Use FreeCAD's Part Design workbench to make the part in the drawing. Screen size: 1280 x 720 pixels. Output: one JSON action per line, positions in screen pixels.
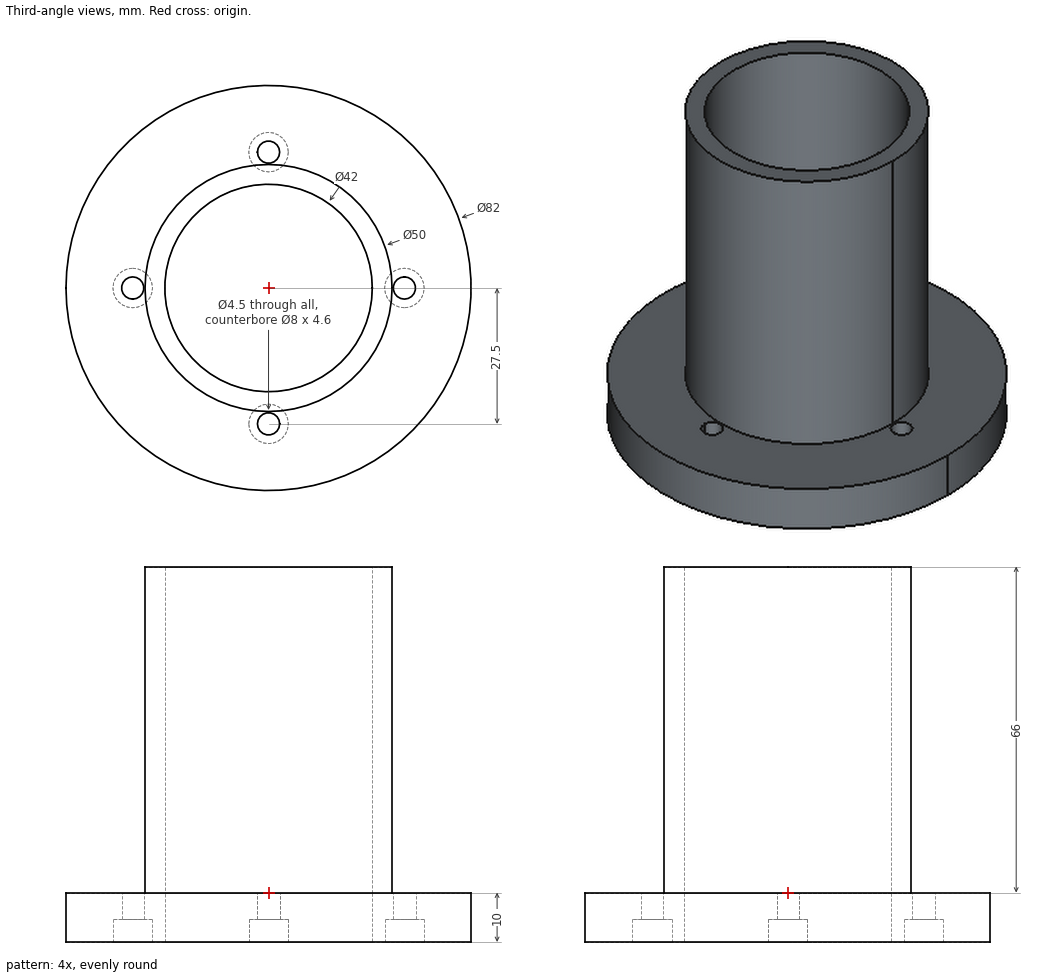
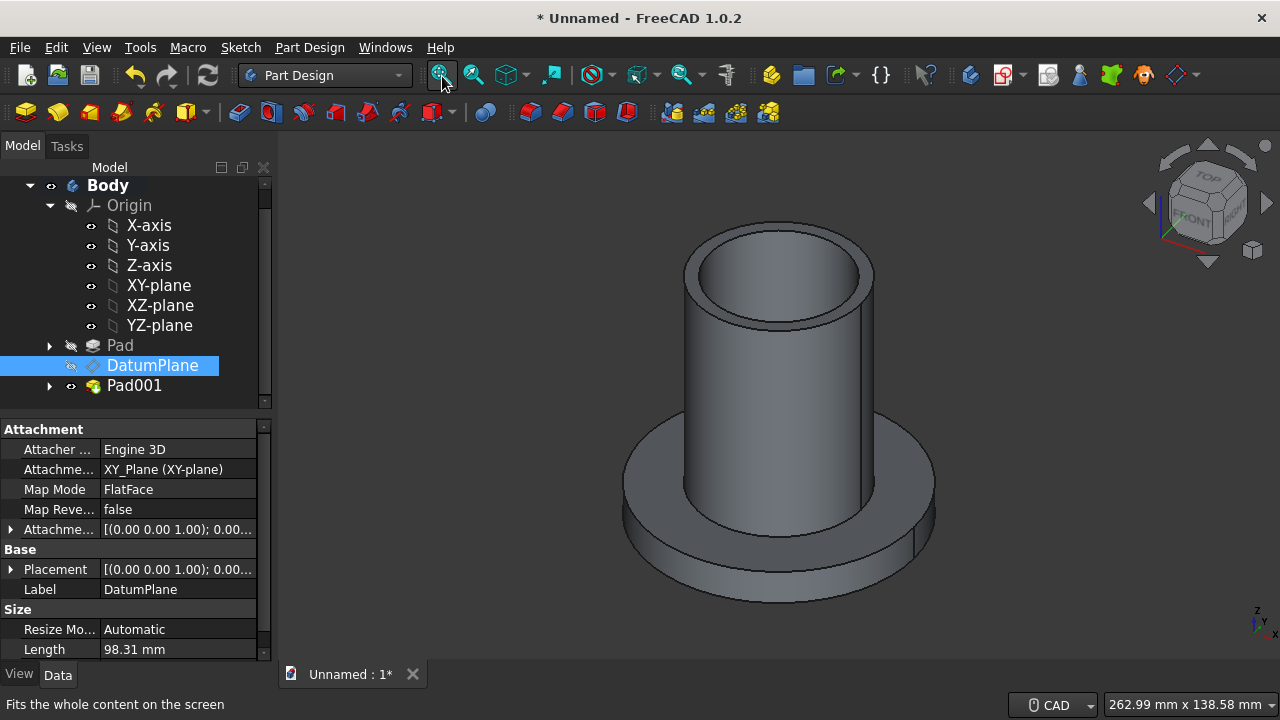
{"action": "key", "text": "5"}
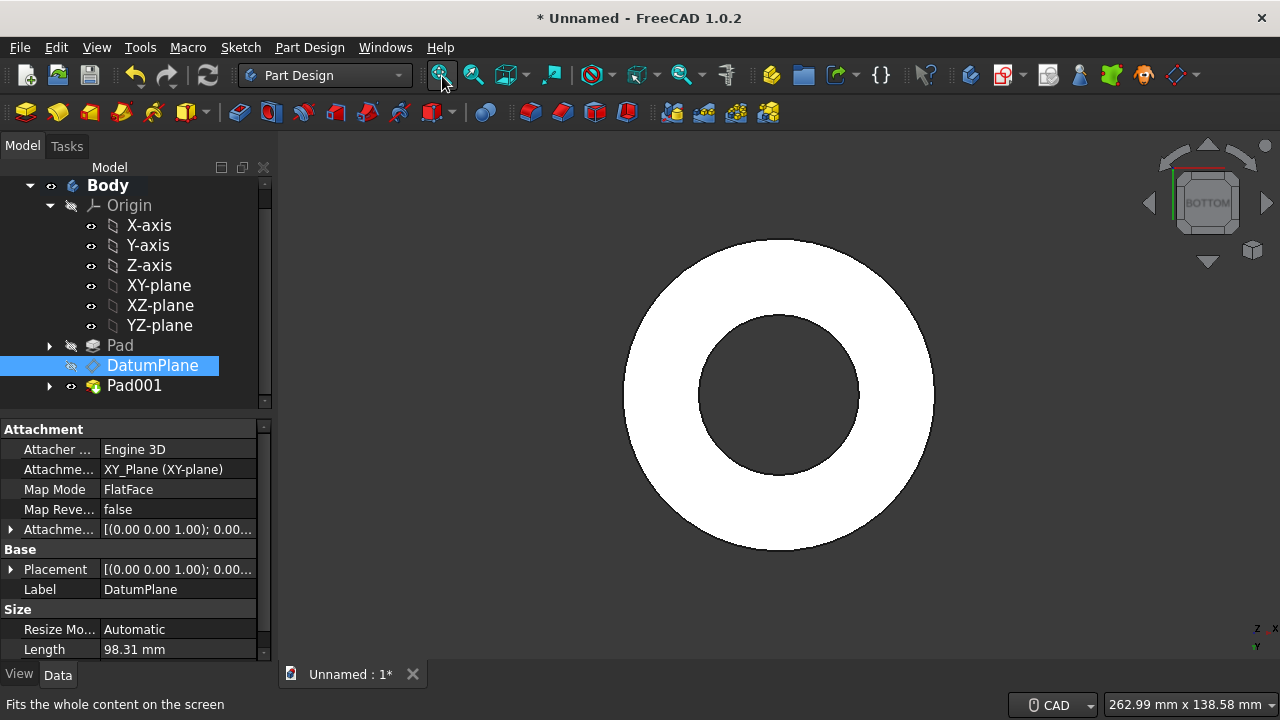
{"action": "left_click", "coordinate": [868, 305]}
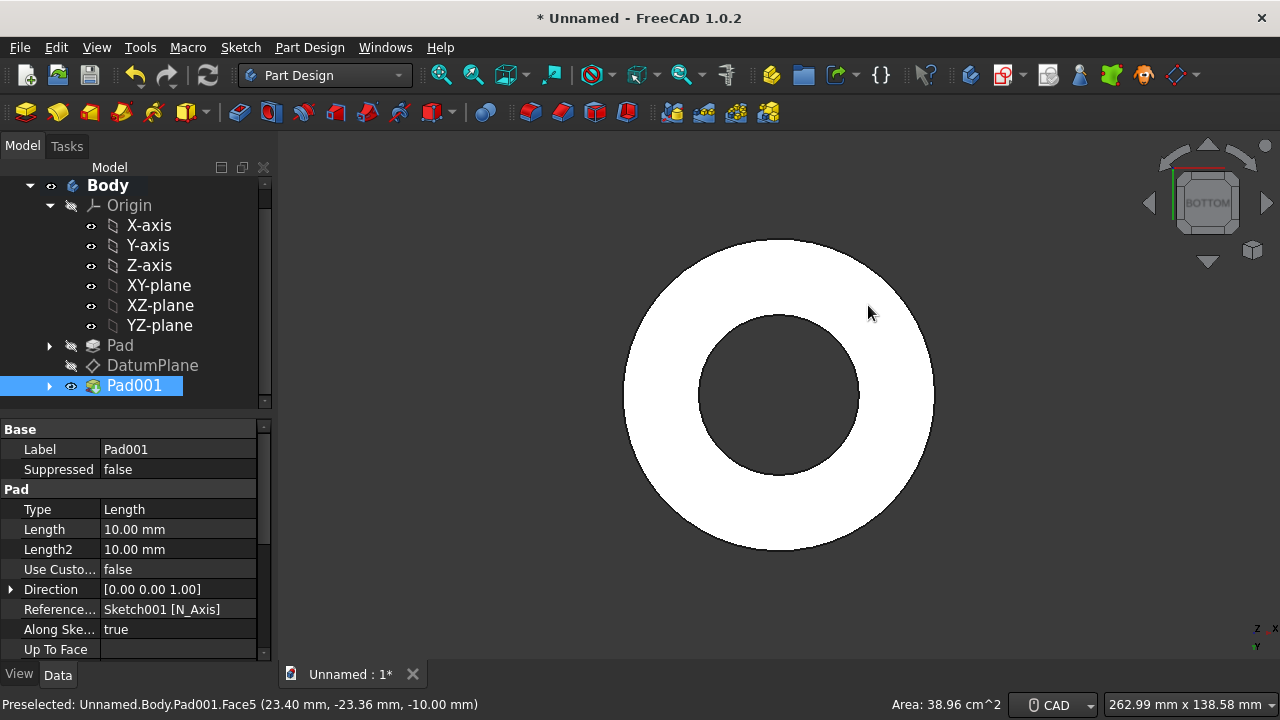
{"action": "left_click", "coordinate": [1004, 76]}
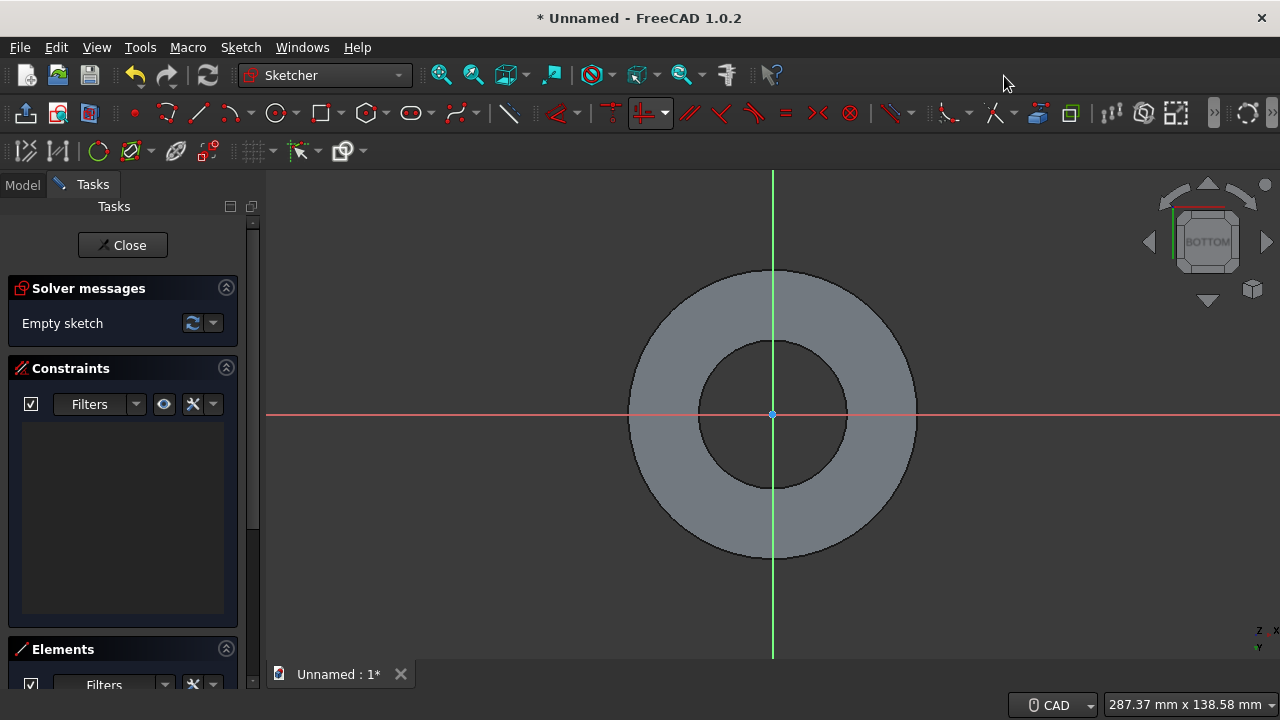
{"action": "scroll", "coordinate": [776, 312], "scroll_direction": "up", "scroll_amount": 15}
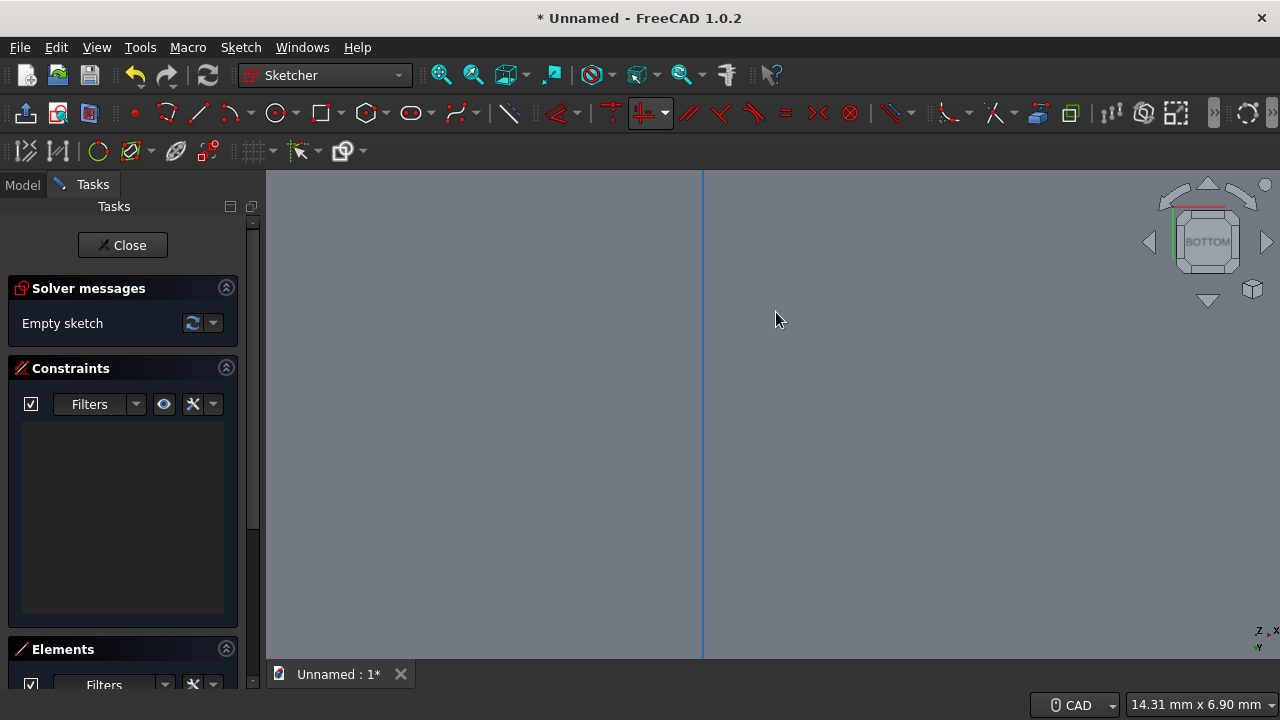
{"action": "key", "text": "g c"}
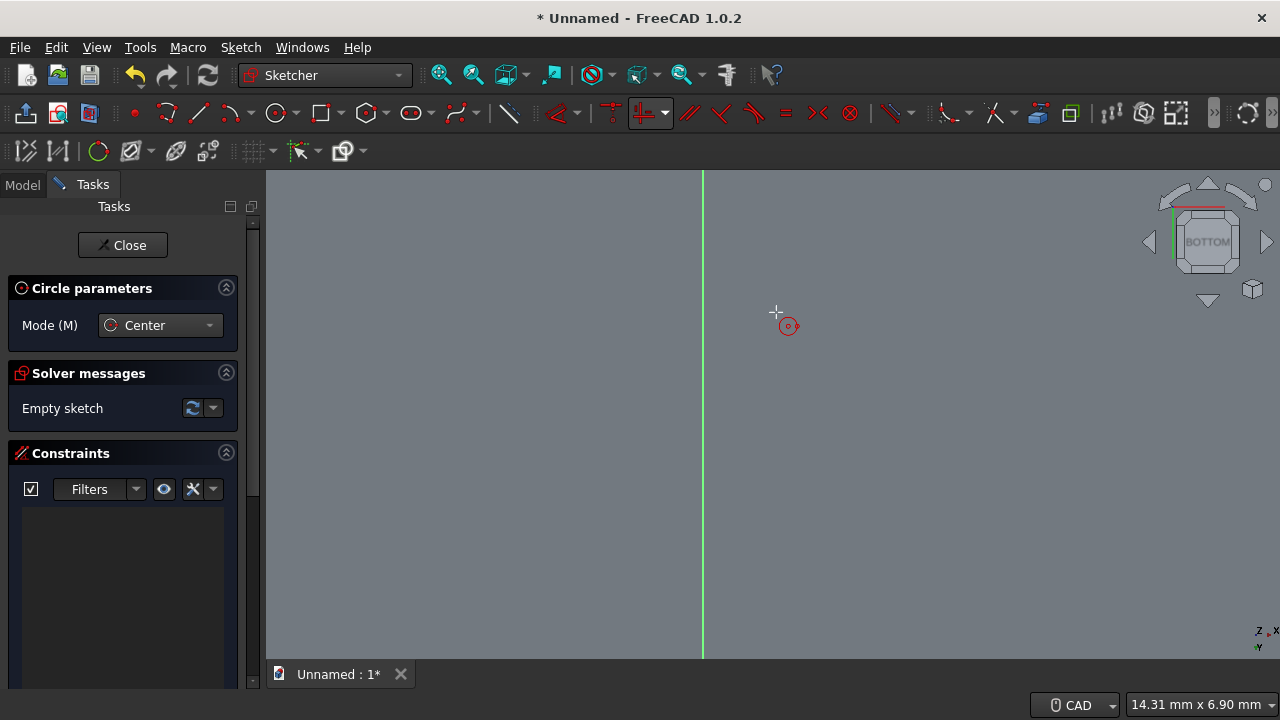
{"action": "left_click", "coordinate": [703, 416]}
{"action": "left_click", "coordinate": [816, 303]}
{"action": "key", "text": "Escape"}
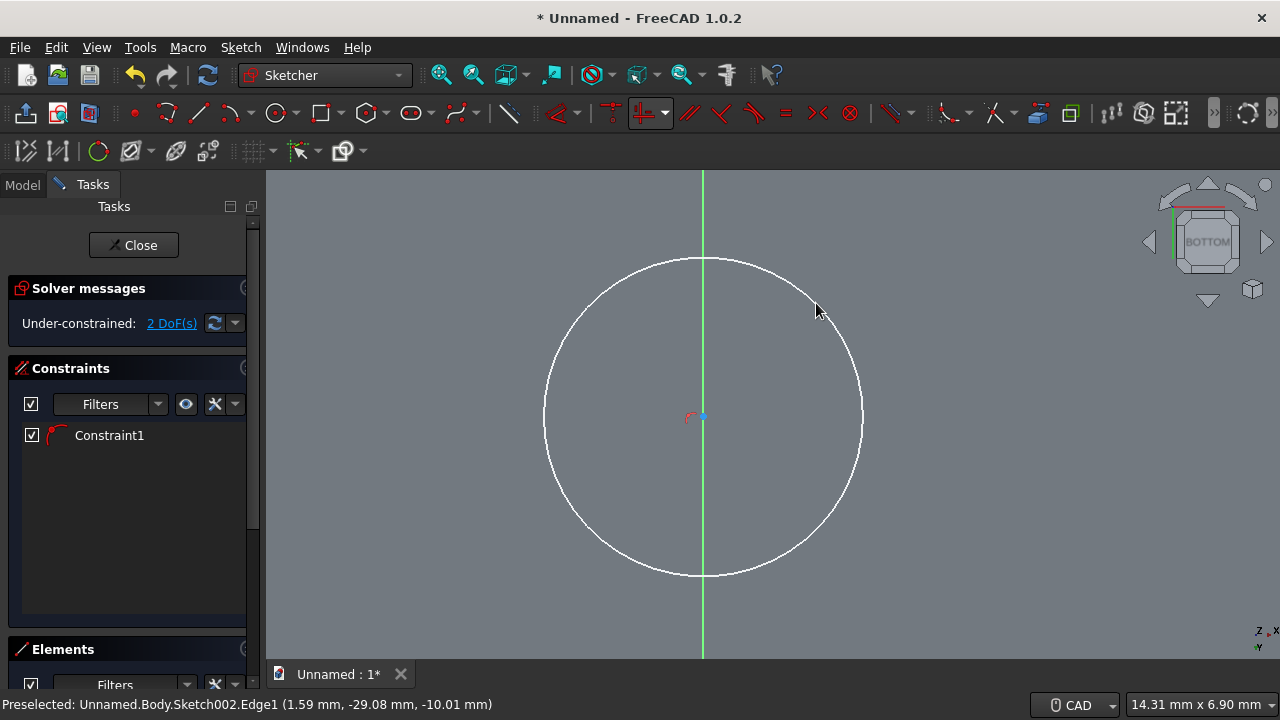
{"action": "left_click", "coordinate": [556, 114]}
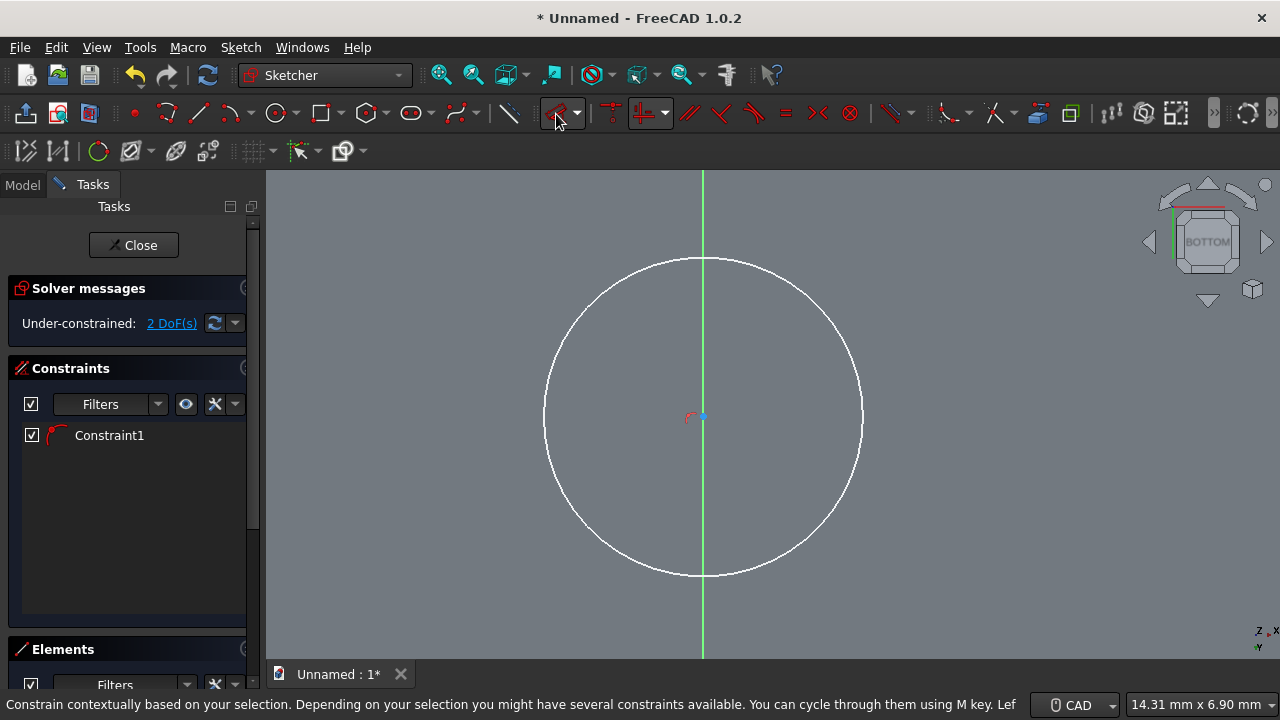
{"action": "left_click", "coordinate": [816, 304]}
{"action": "left_click", "coordinate": [839, 281]}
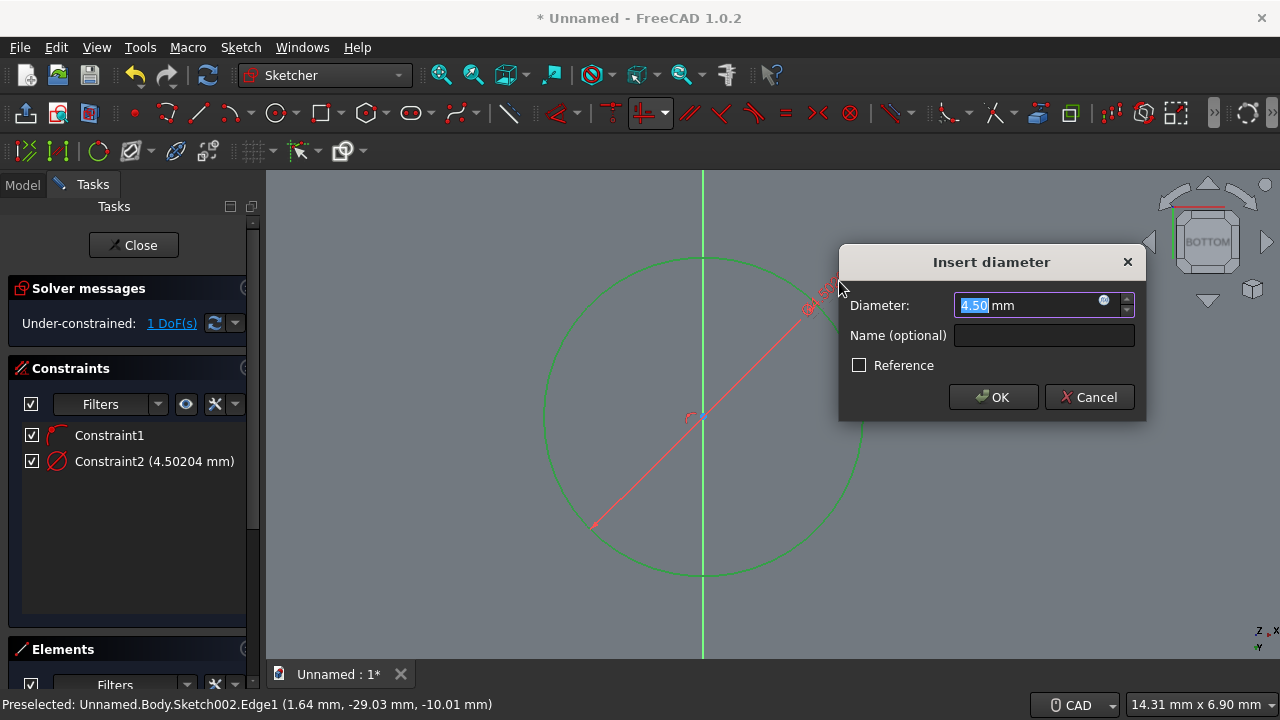
{"action": "type", "text": "4.5"}
{"action": "key", "text": "Return"}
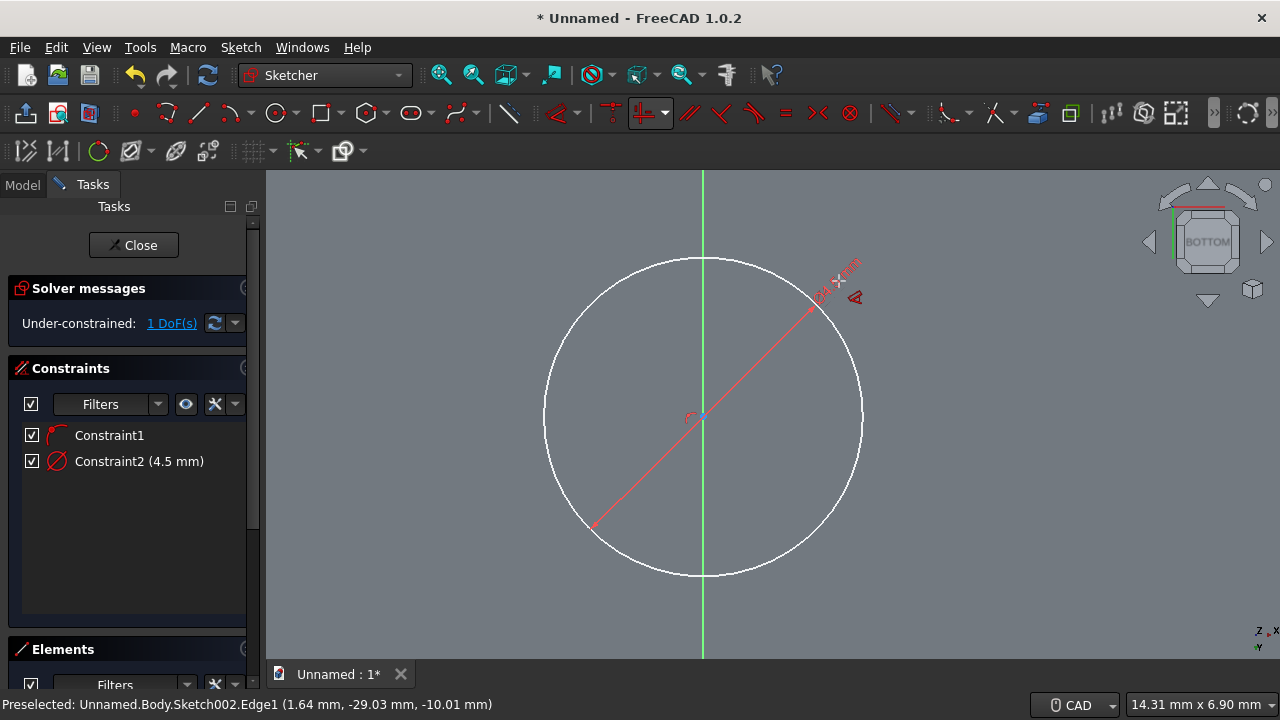
{"action": "left_click", "coordinate": [703, 417]}
{"action": "left_click", "coordinate": [737, 524]}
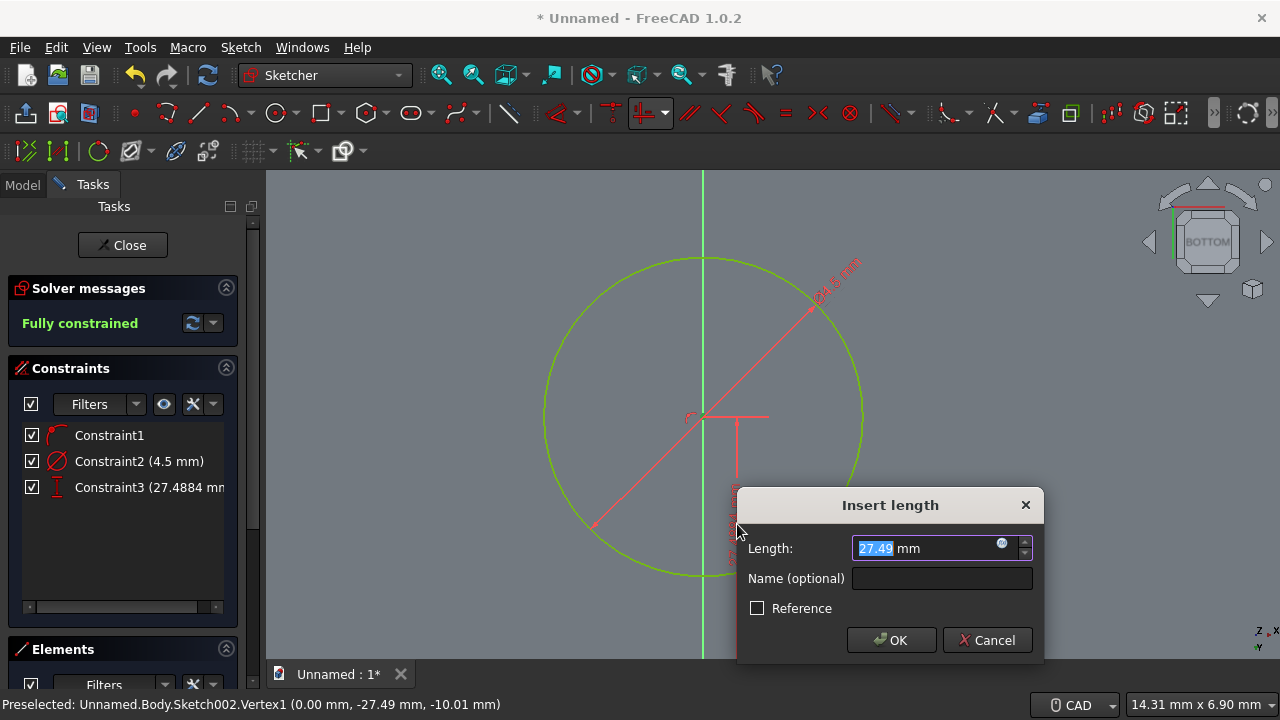
{"action": "type", "text": "27.5"}
{"action": "key", "text": "Return"}
{"action": "key", "text": "Escape"}